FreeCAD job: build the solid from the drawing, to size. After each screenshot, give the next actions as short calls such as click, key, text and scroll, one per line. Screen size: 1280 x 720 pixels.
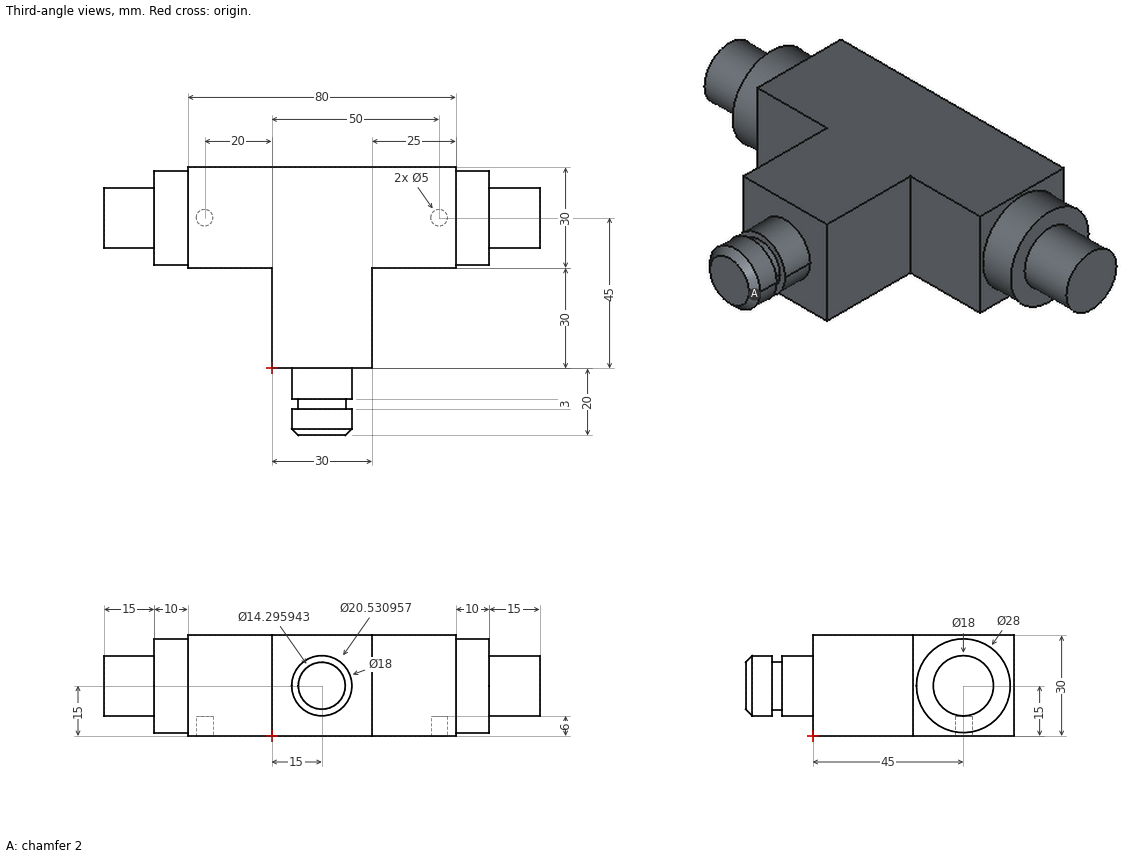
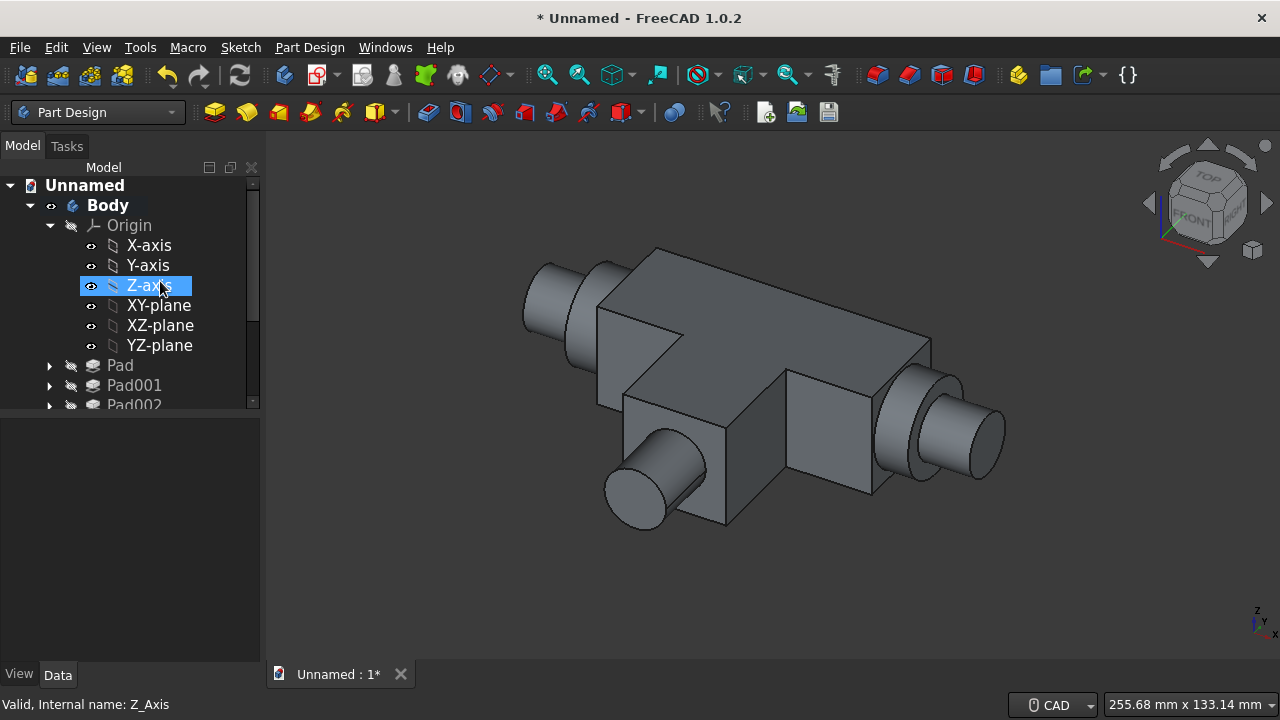
click(136, 326)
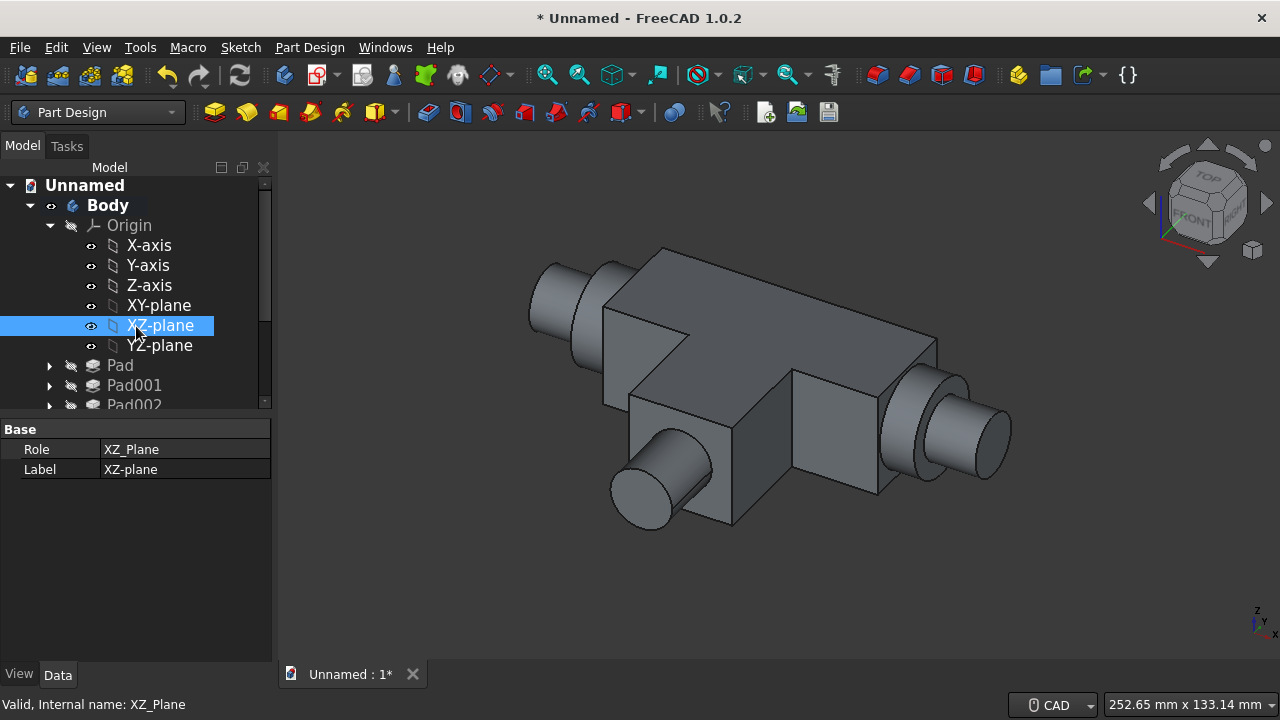
click(490, 76)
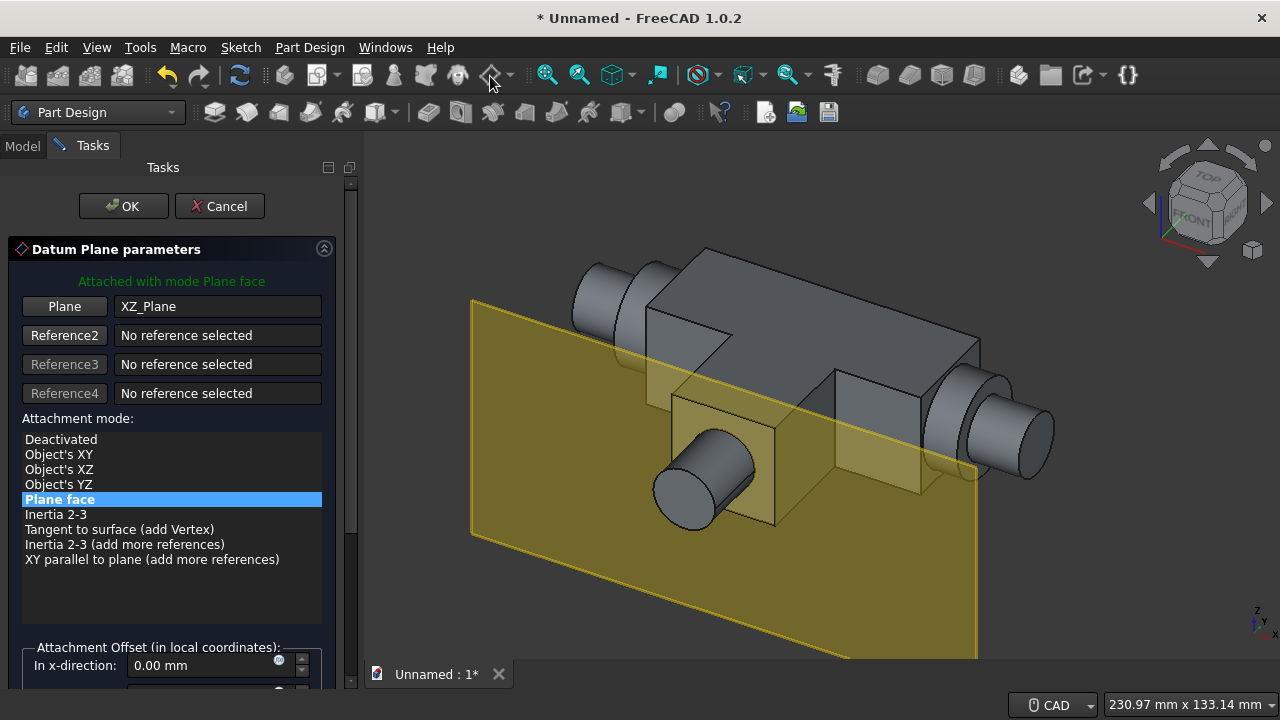
scroll(351, 432, down, 2)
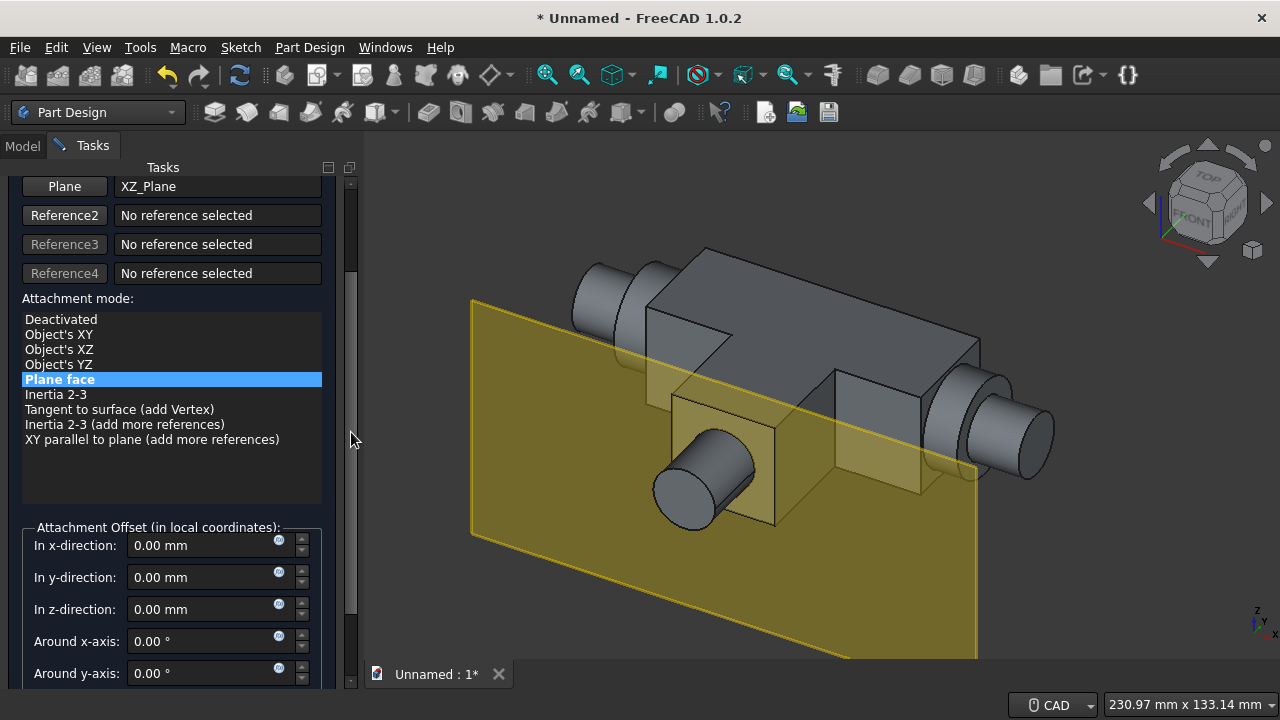
triple_click(210, 609)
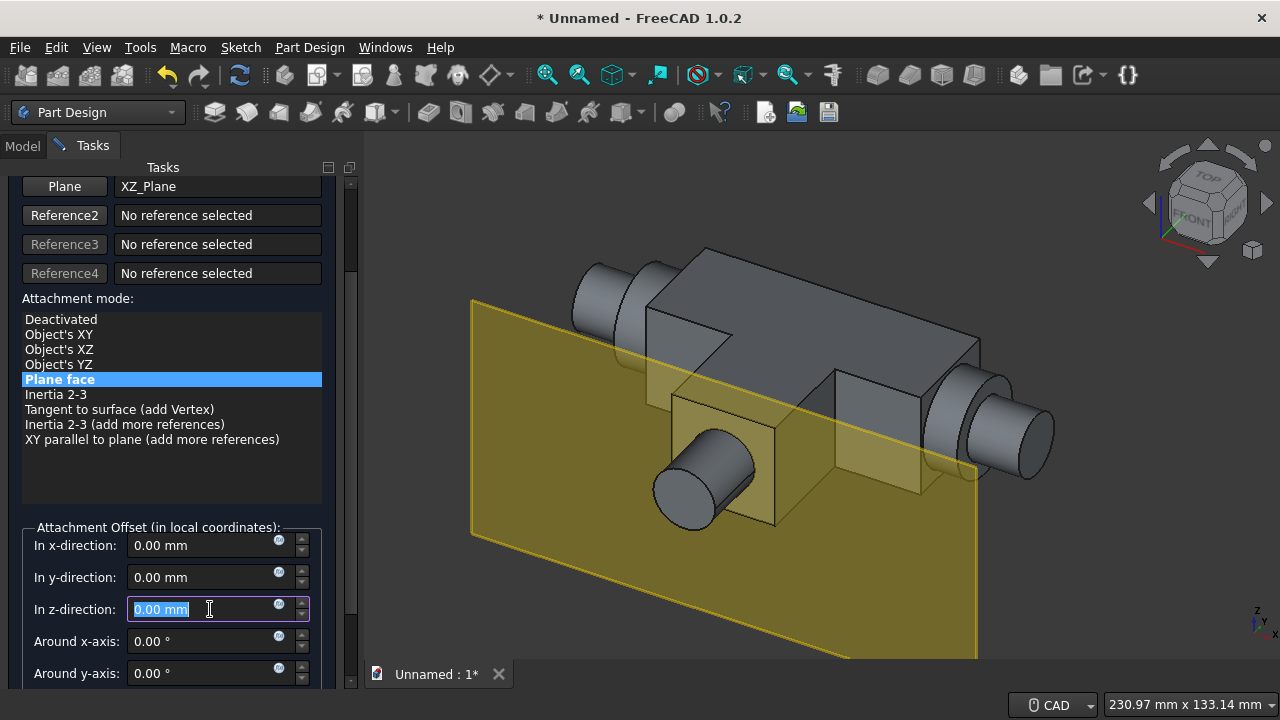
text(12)
key(Tab)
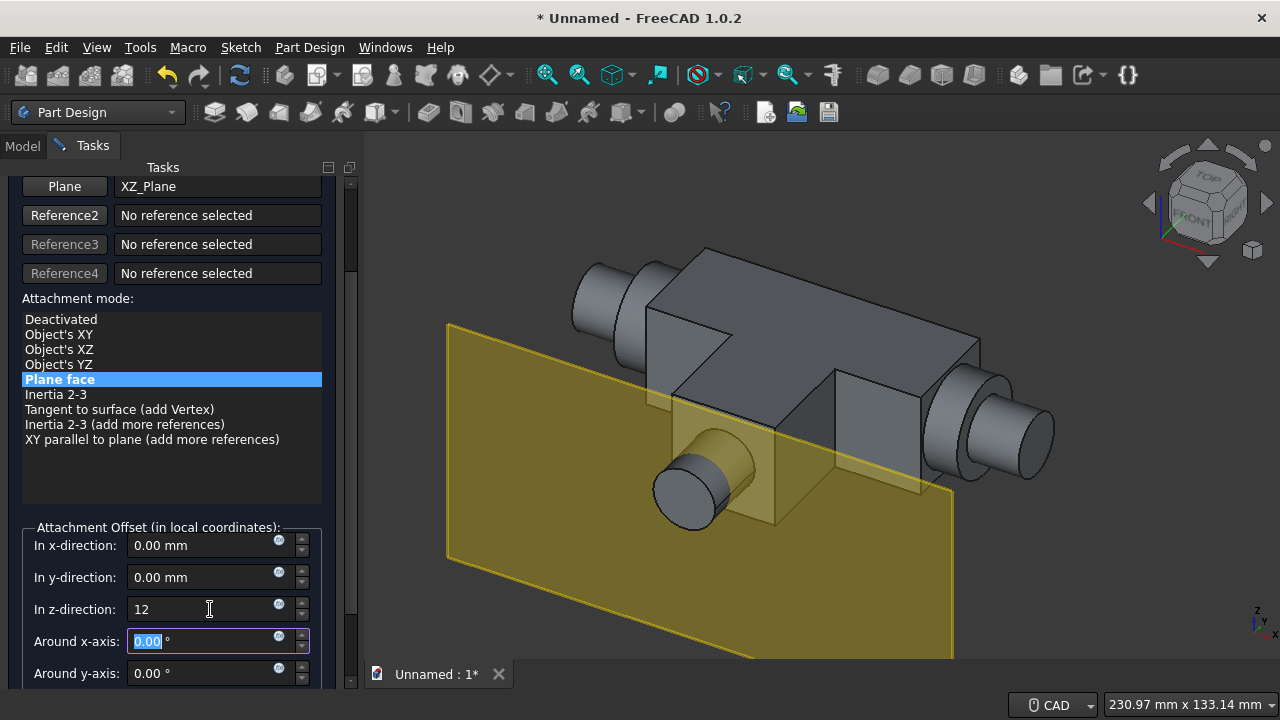
scroll(351, 432, up, 3)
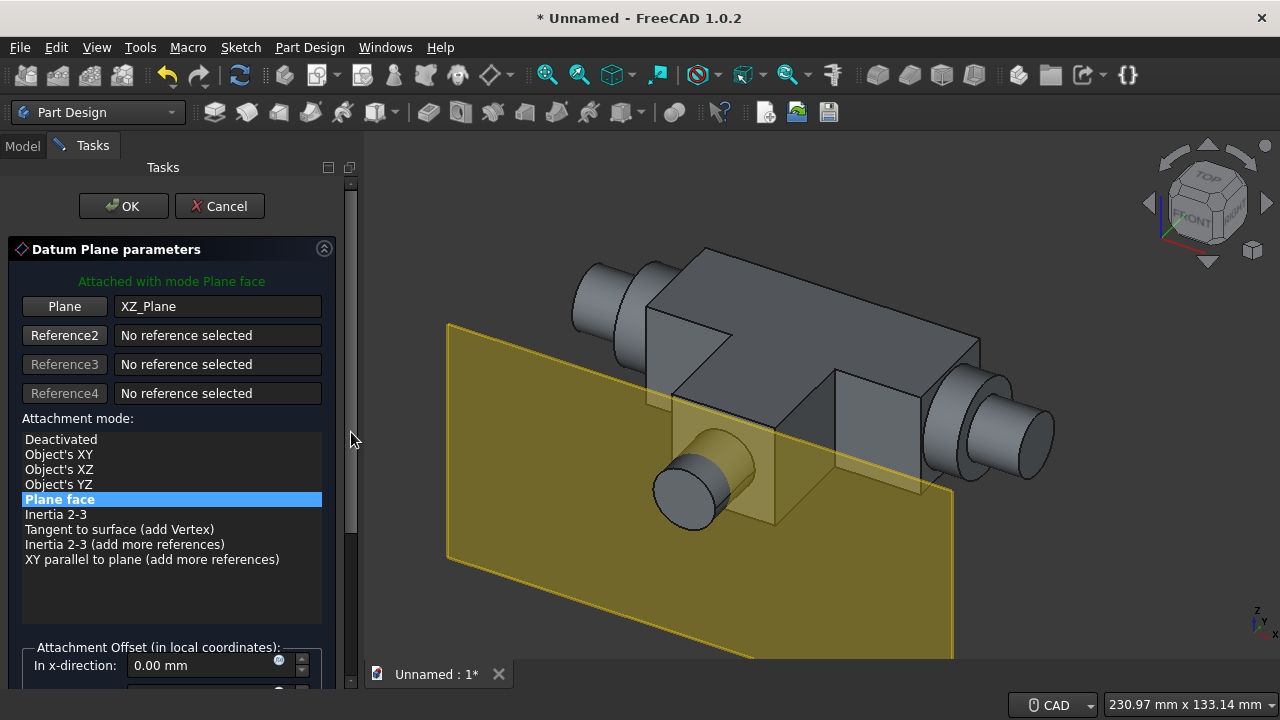
click(124, 206)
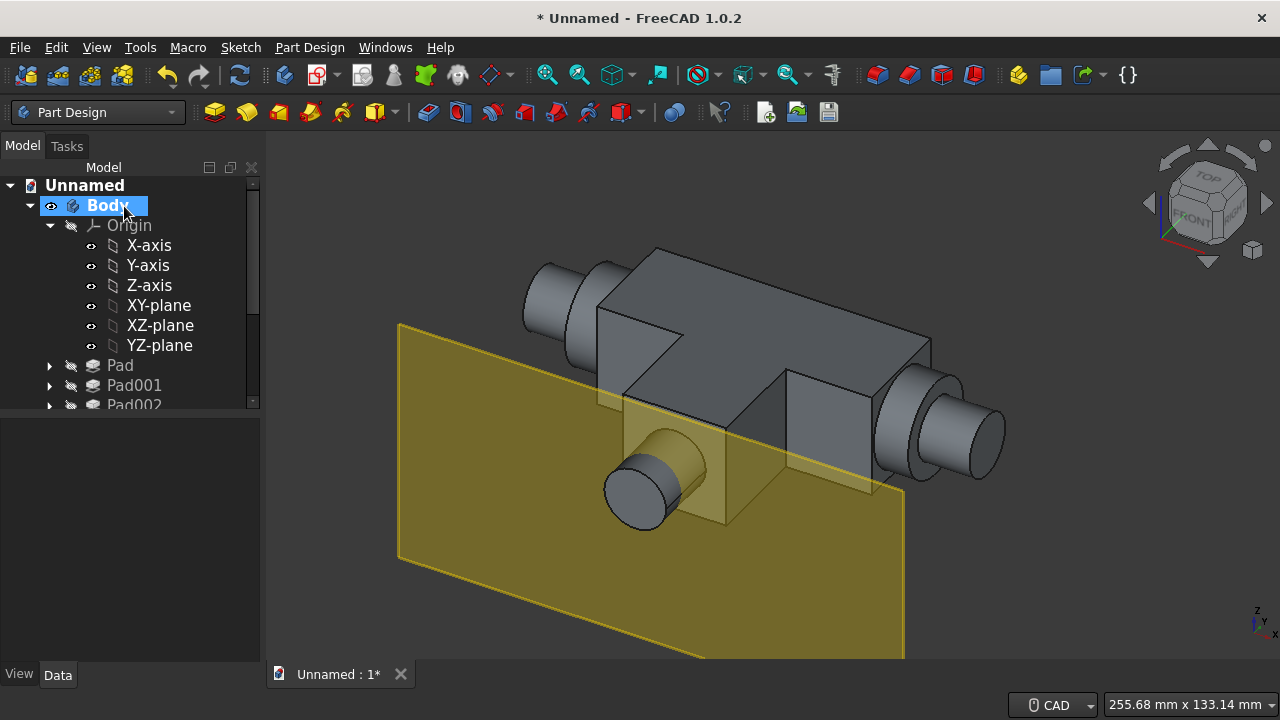
scroll(100, 301, down, 3)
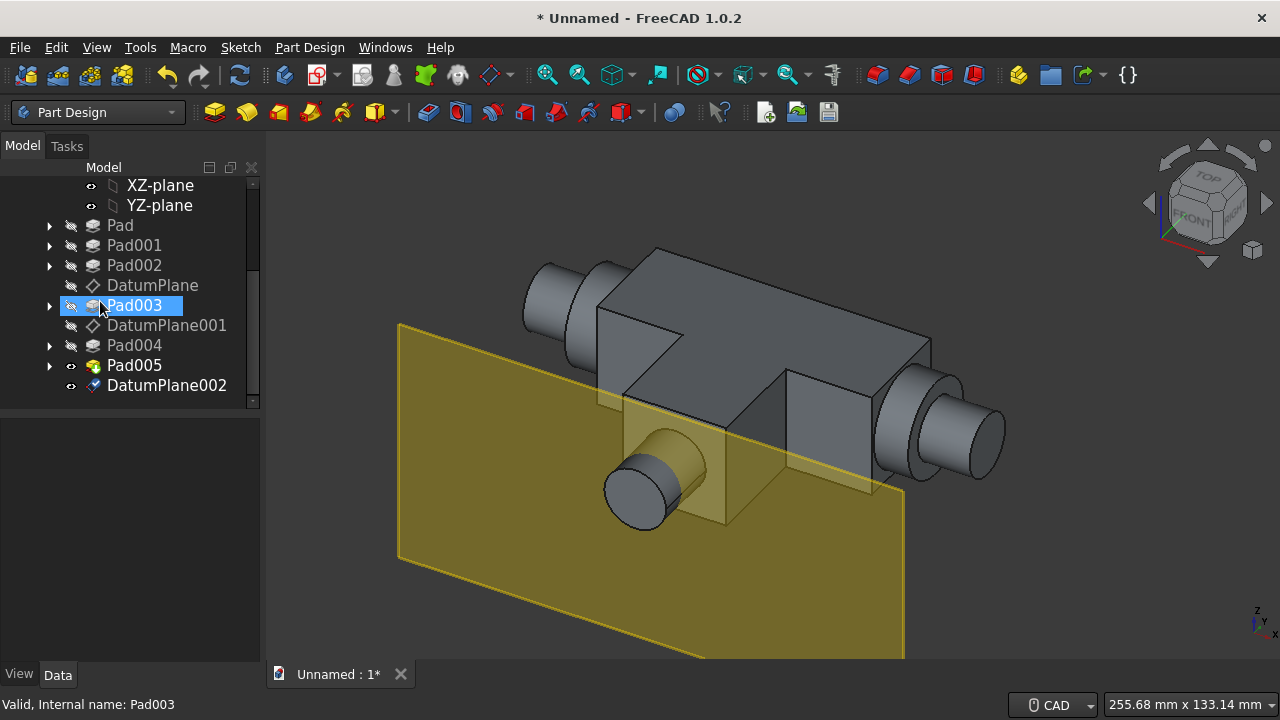
click(116, 386)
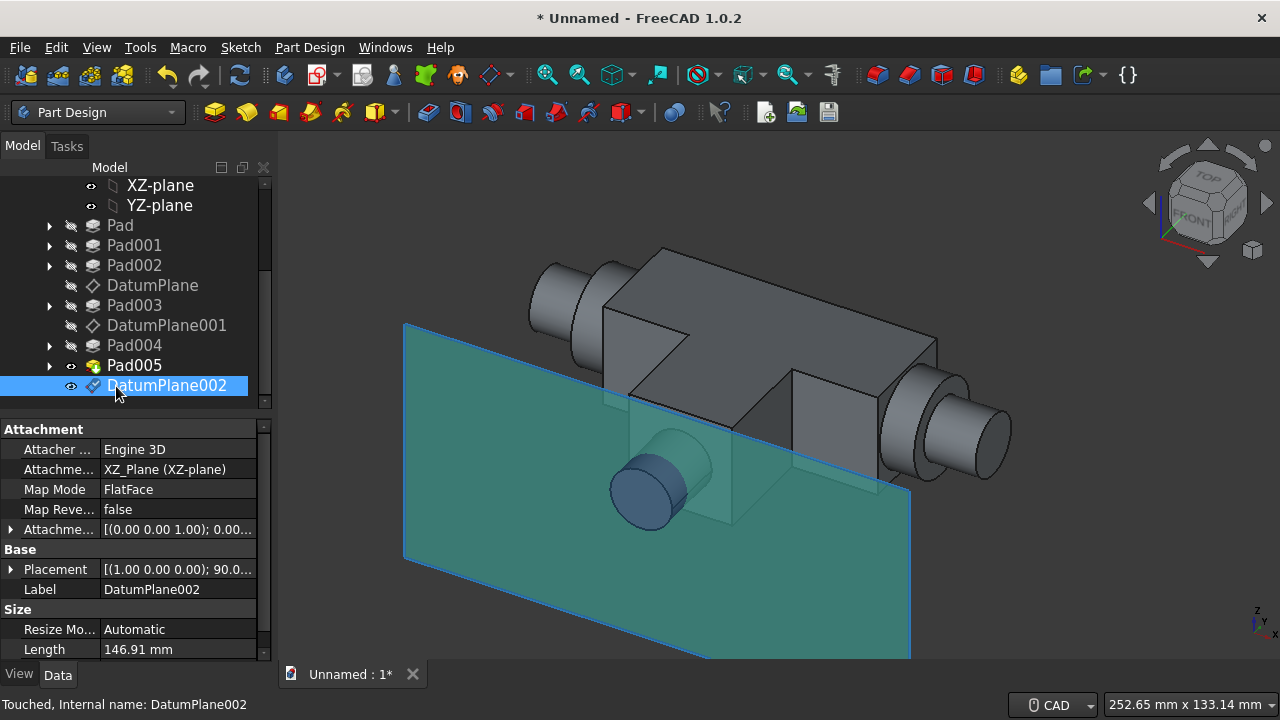
click(318, 76)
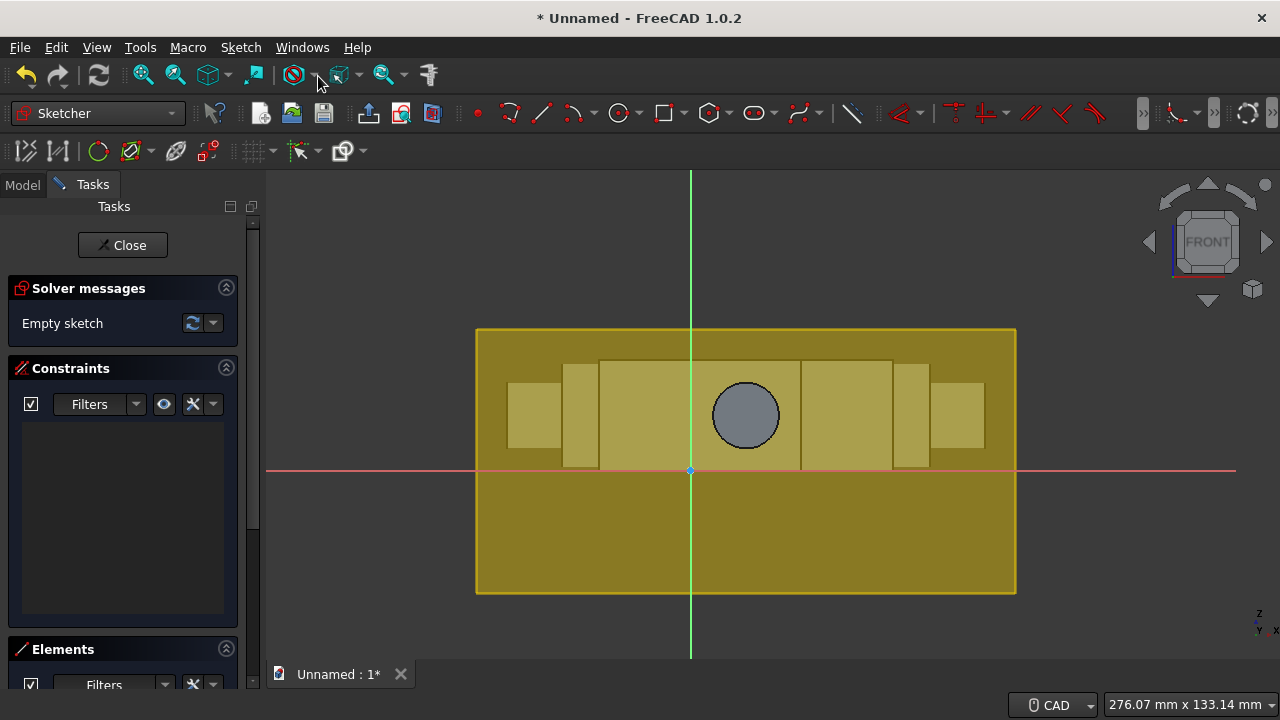
key(q)
key(s)